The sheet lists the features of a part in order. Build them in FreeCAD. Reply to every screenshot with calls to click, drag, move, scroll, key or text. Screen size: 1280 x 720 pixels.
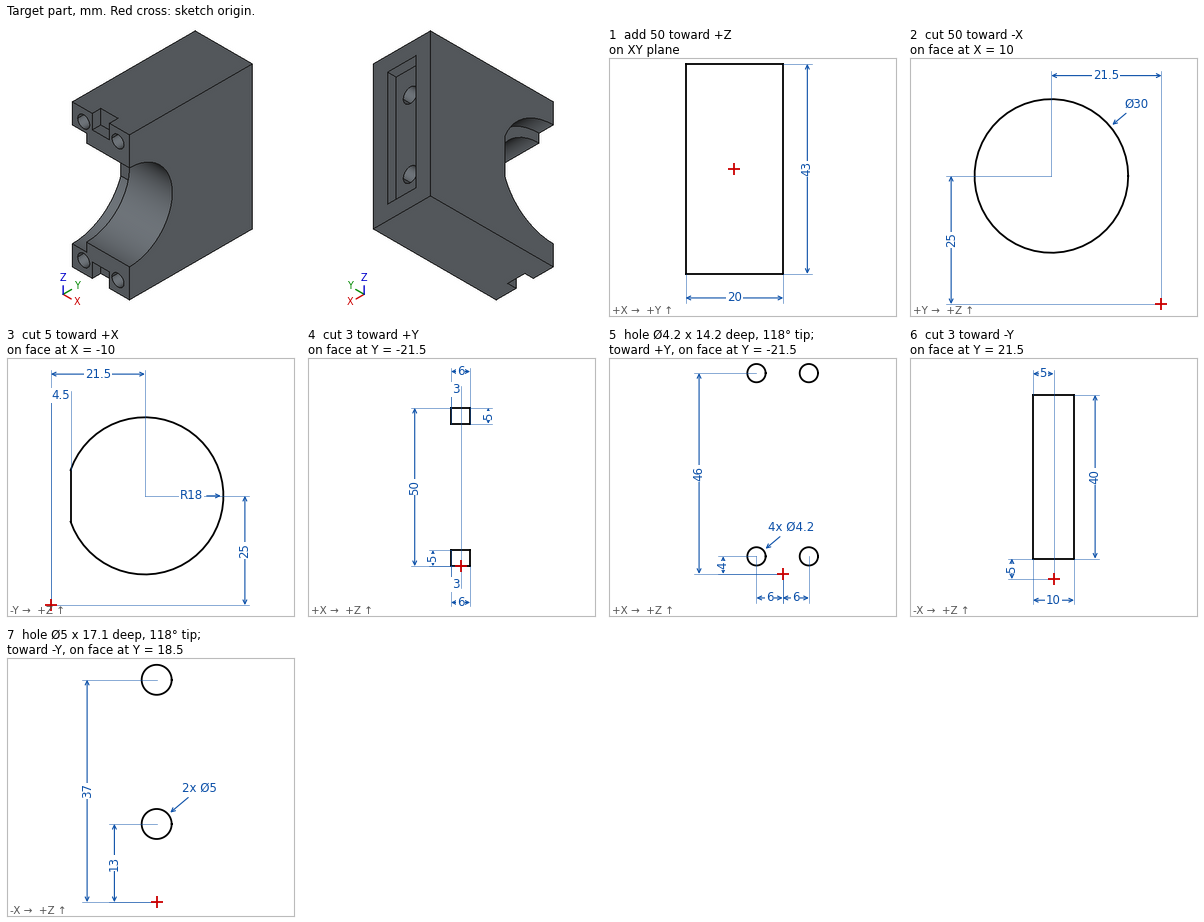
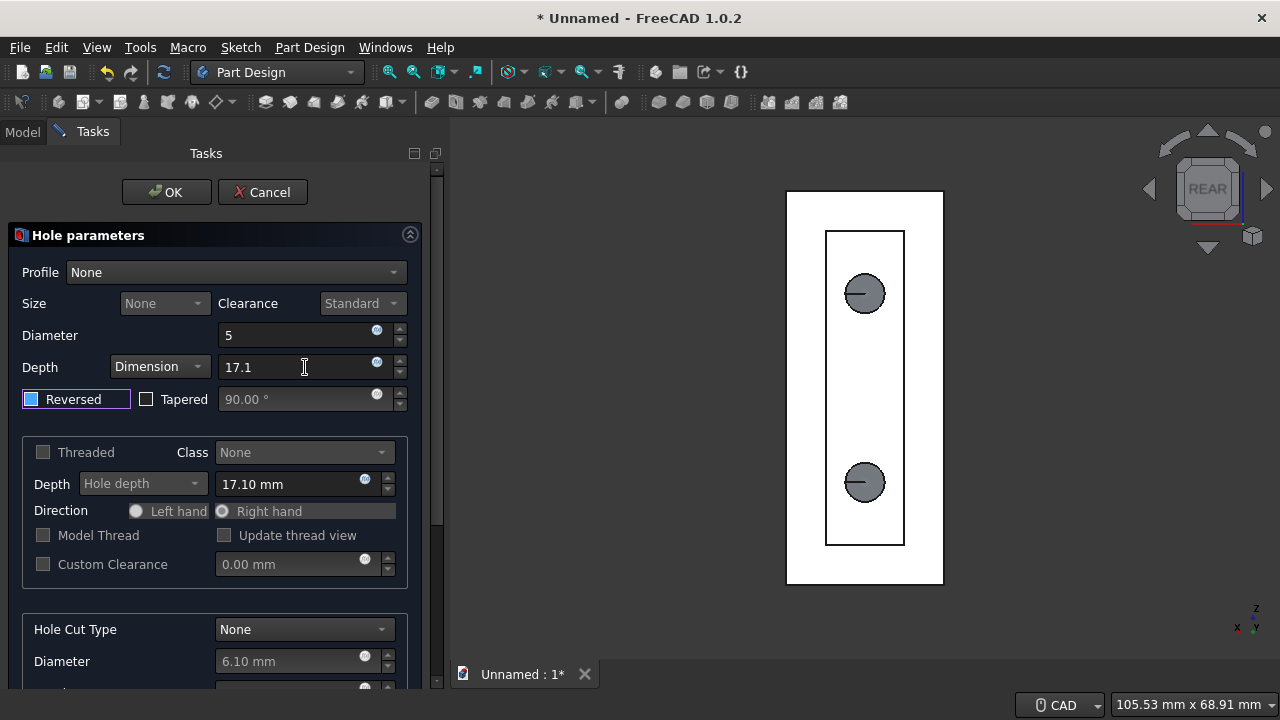
click(167, 192)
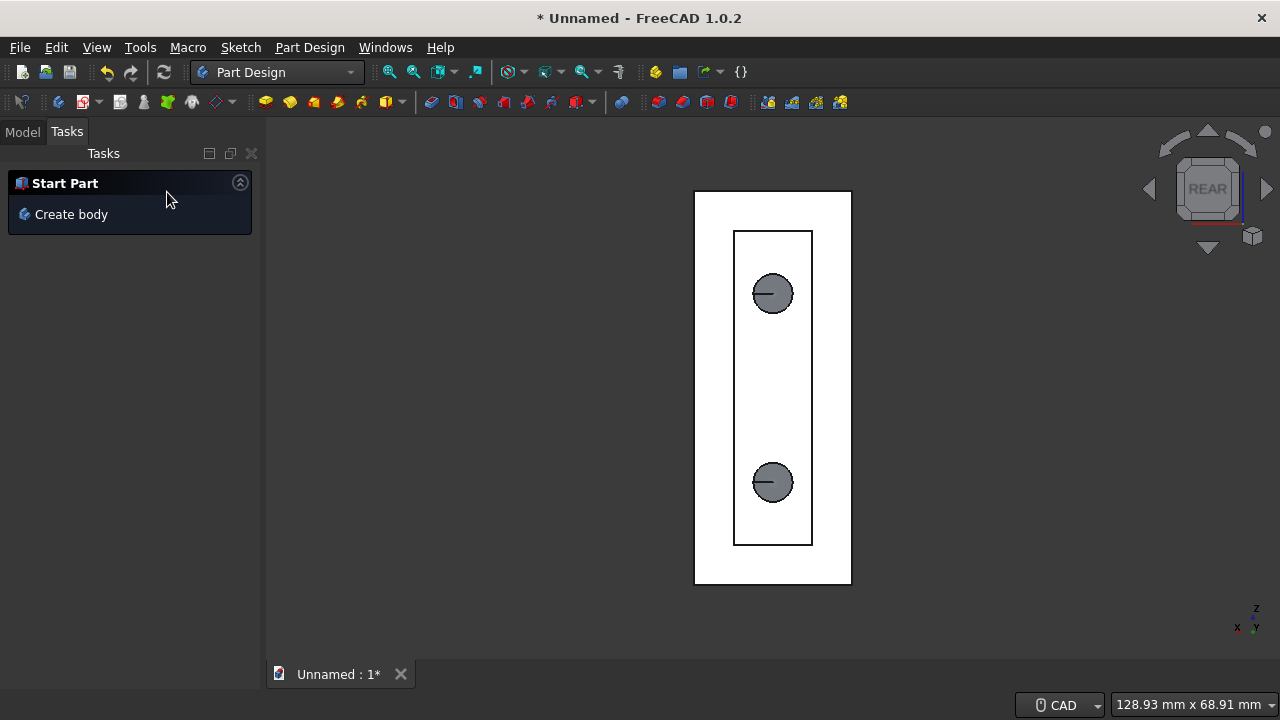
key(0)